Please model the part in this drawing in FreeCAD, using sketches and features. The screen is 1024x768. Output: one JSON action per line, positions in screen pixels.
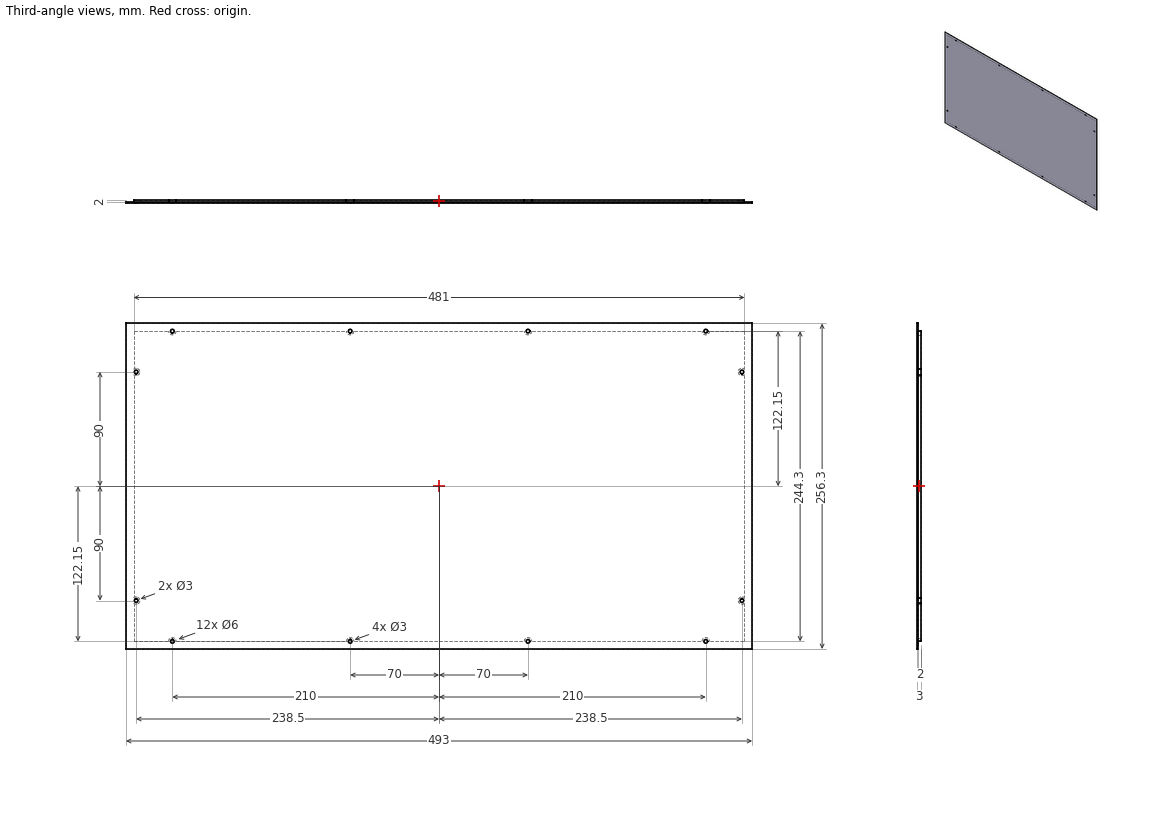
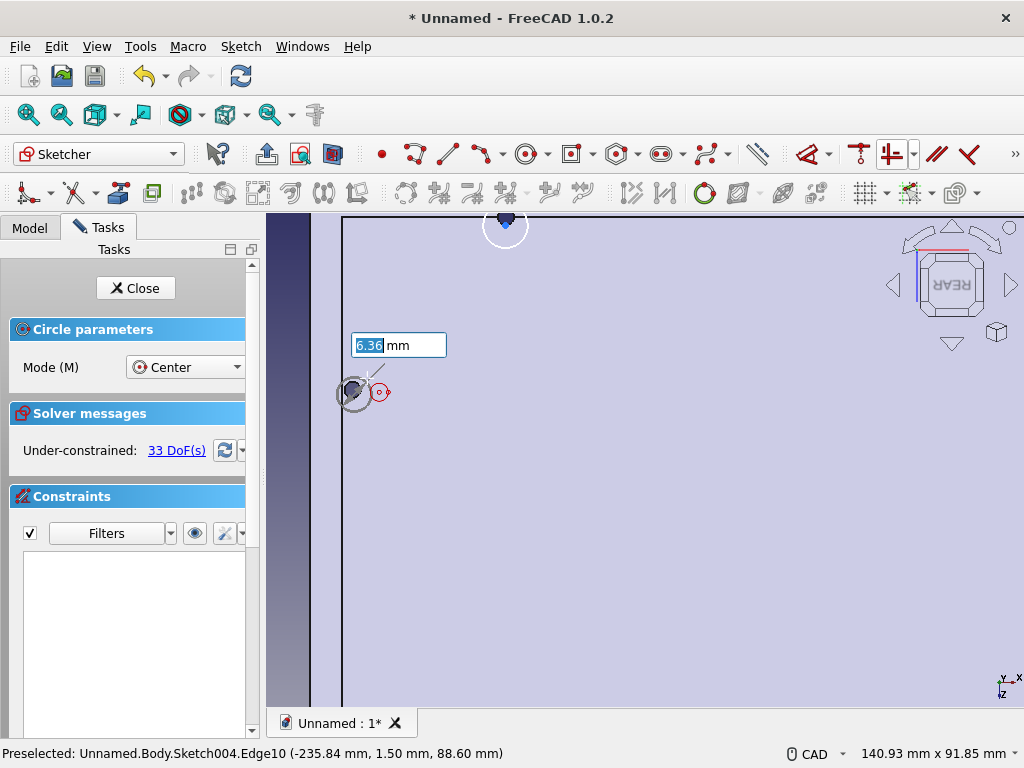
{"action": "left_click", "coordinate": [364, 378]}
{"action": "key", "text": "Escape"}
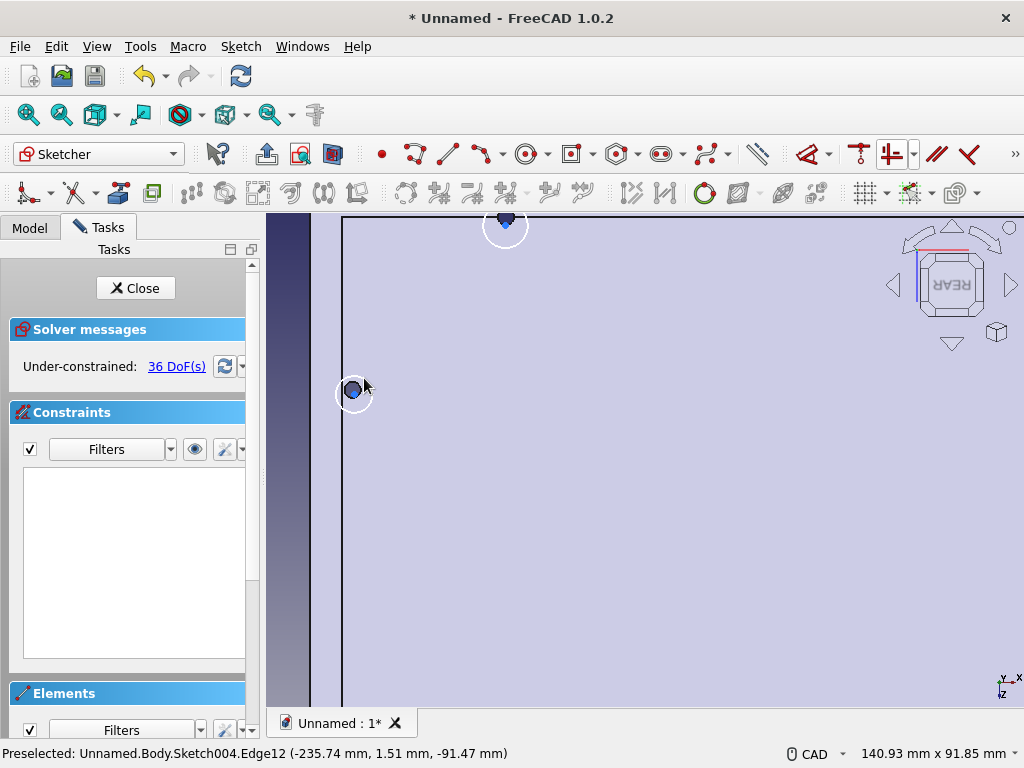
{"action": "left_click", "coordinate": [490, 241]}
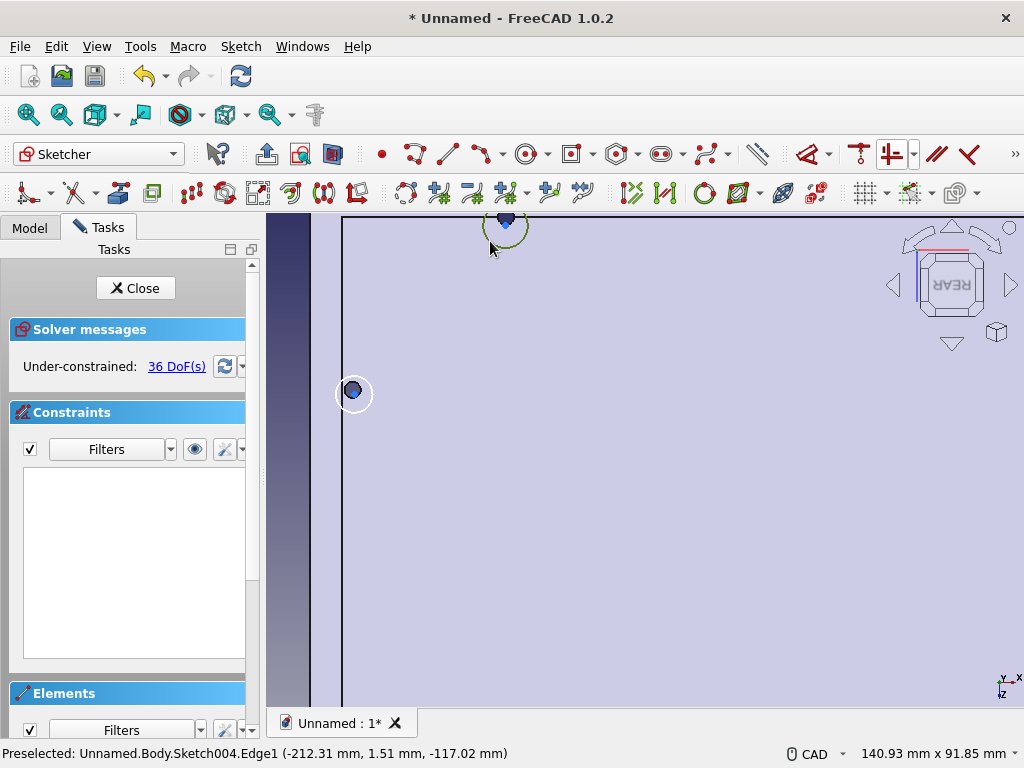
{"action": "scroll", "coordinate": [367, 378], "scroll_direction": "down", "scroll_amount": 9}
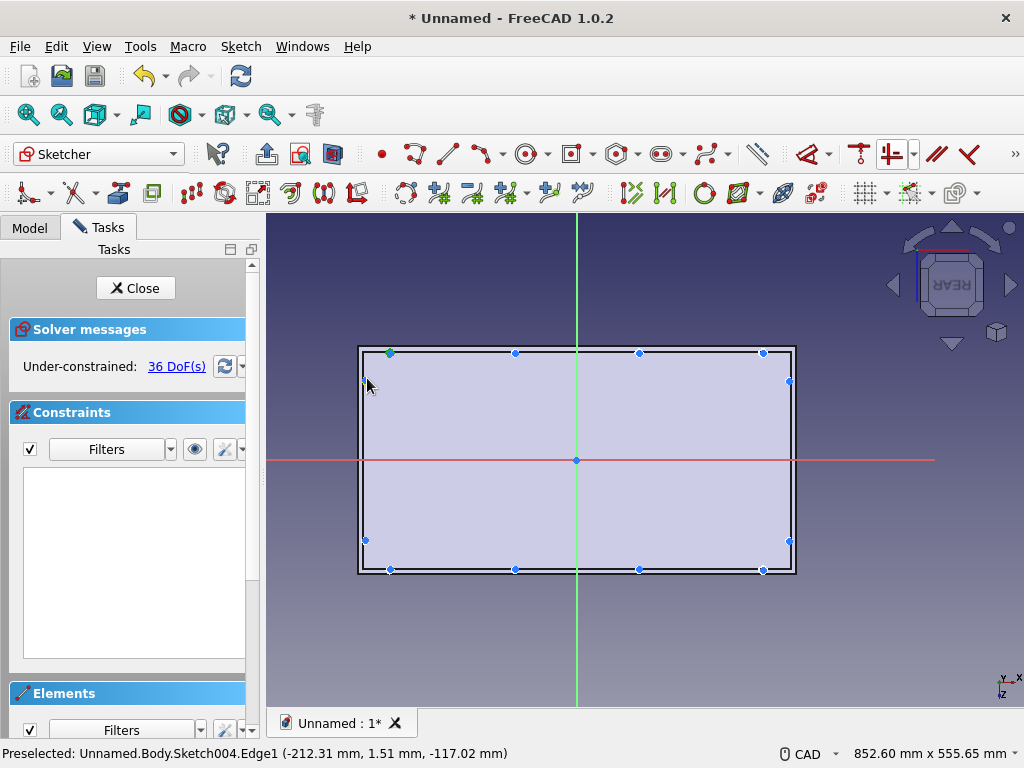
{"action": "scroll", "coordinate": [517, 351], "scroll_direction": "up", "scroll_amount": 7}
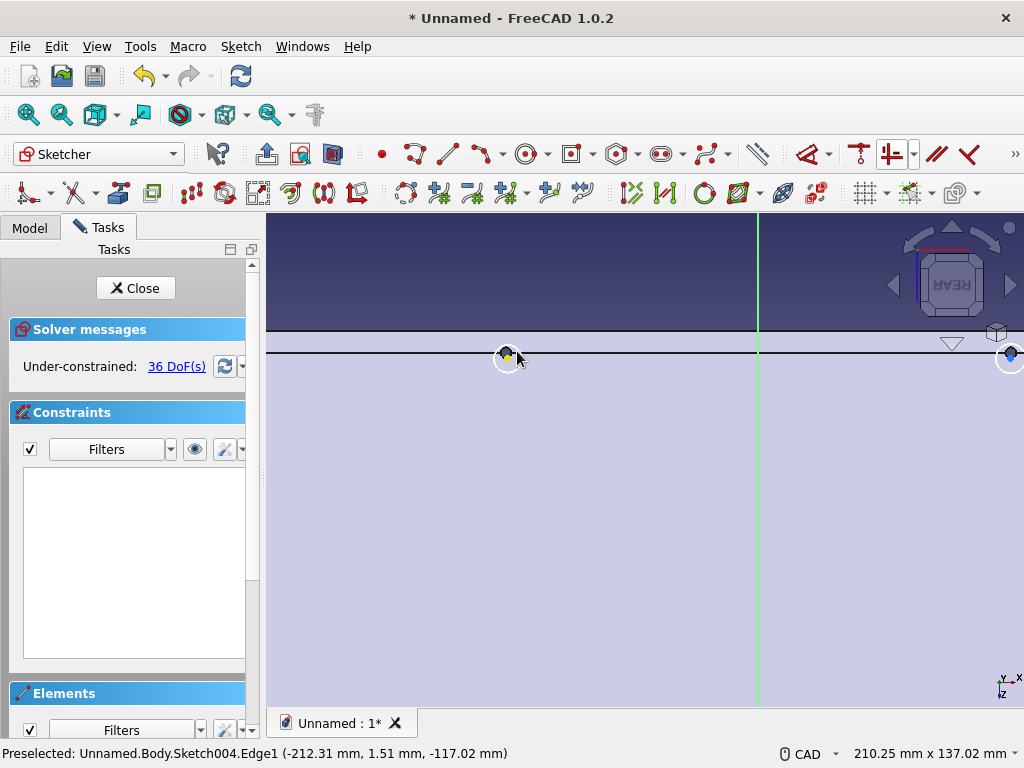
{"action": "left_click", "coordinate": [518, 349]}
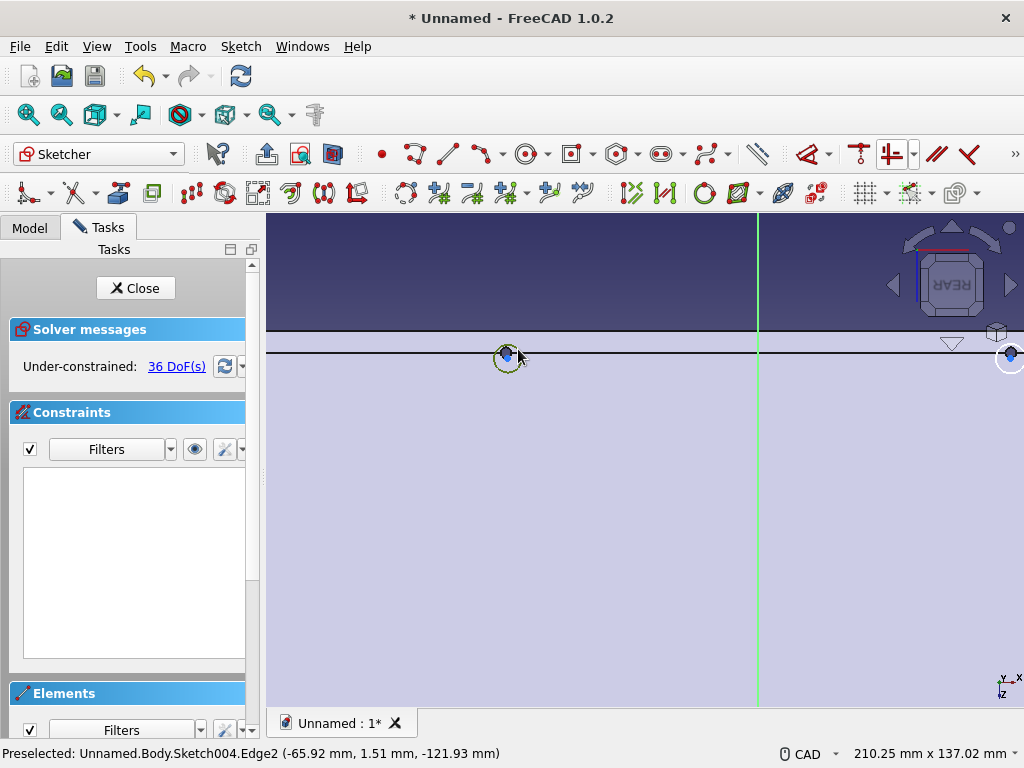
{"action": "scroll", "coordinate": [517, 351], "scroll_direction": "down", "scroll_amount": 7}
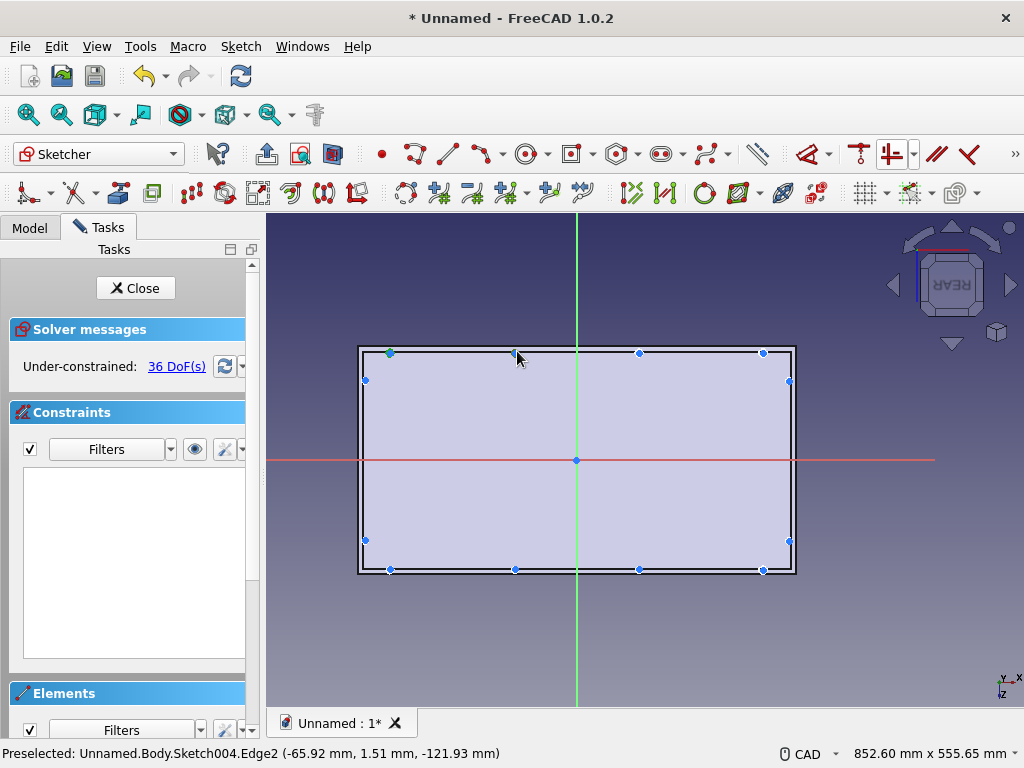
{"action": "scroll", "coordinate": [642, 351], "scroll_direction": "up", "scroll_amount": 7}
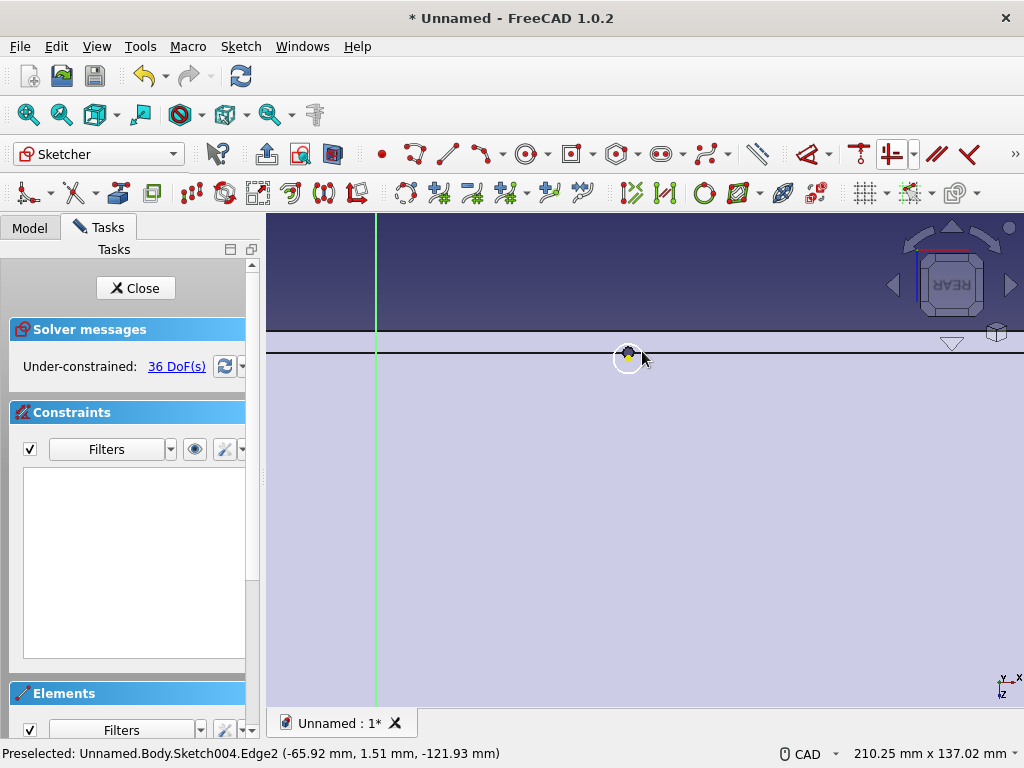
{"action": "left_click", "coordinate": [639, 348]}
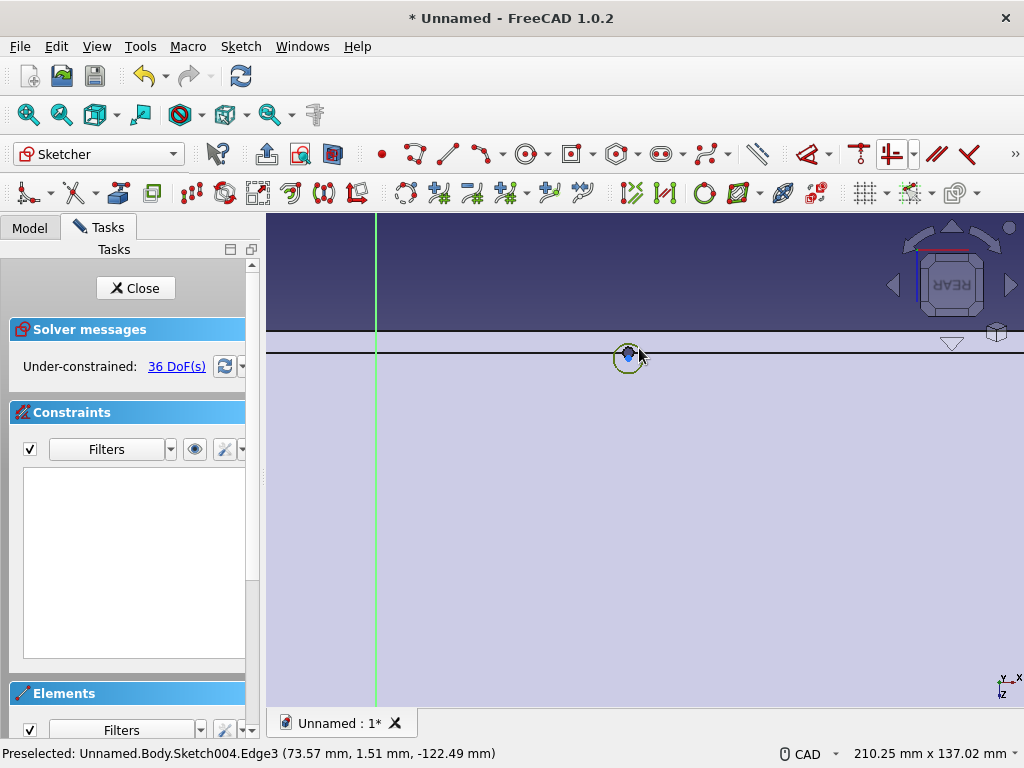
{"action": "scroll", "coordinate": [642, 351], "scroll_direction": "down", "scroll_amount": 7}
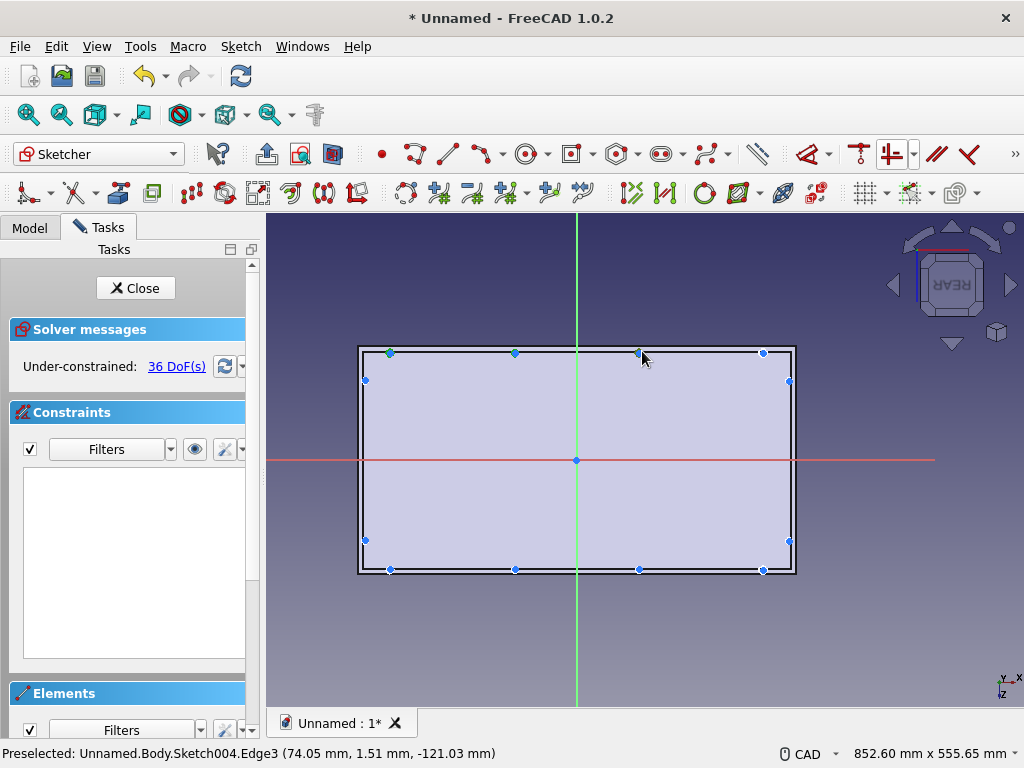
{"action": "scroll", "coordinate": [766, 350], "scroll_direction": "up", "scroll_amount": 7}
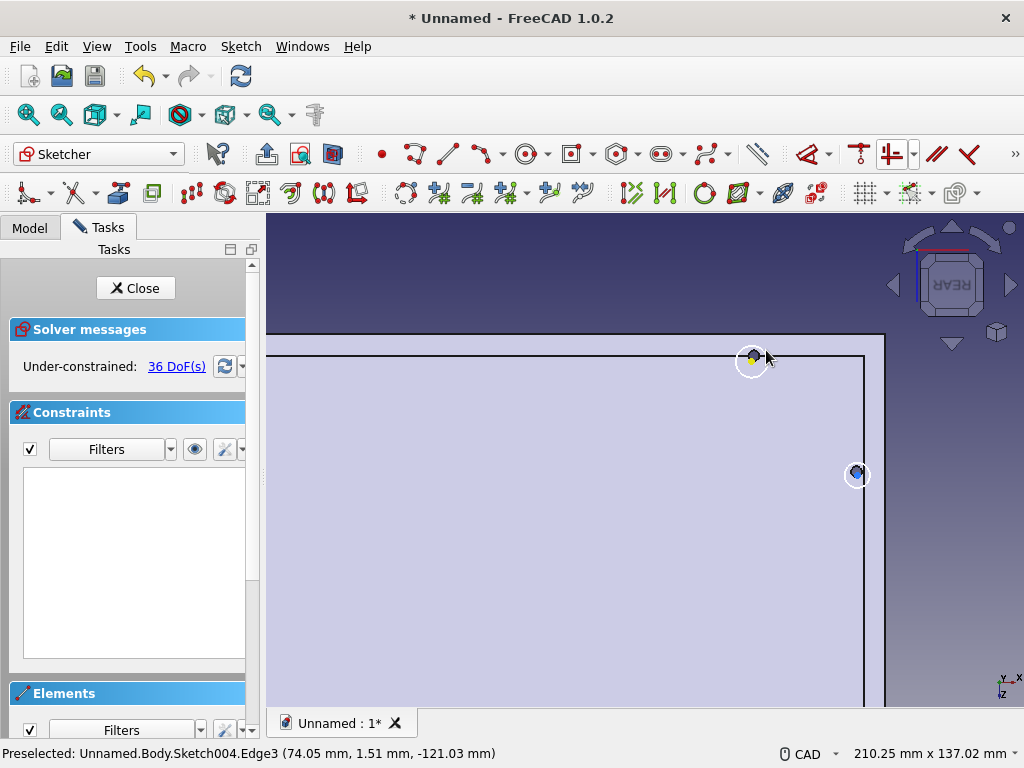
{"action": "left_click", "coordinate": [763, 351]}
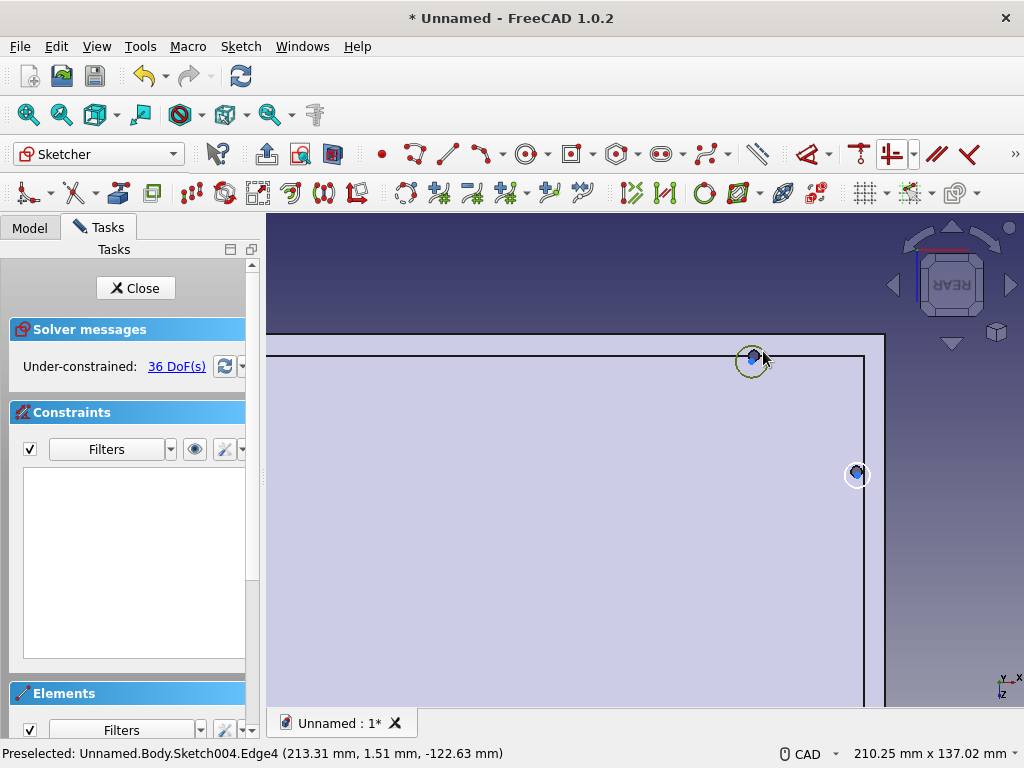
{"action": "left_click", "coordinate": [848, 466]}